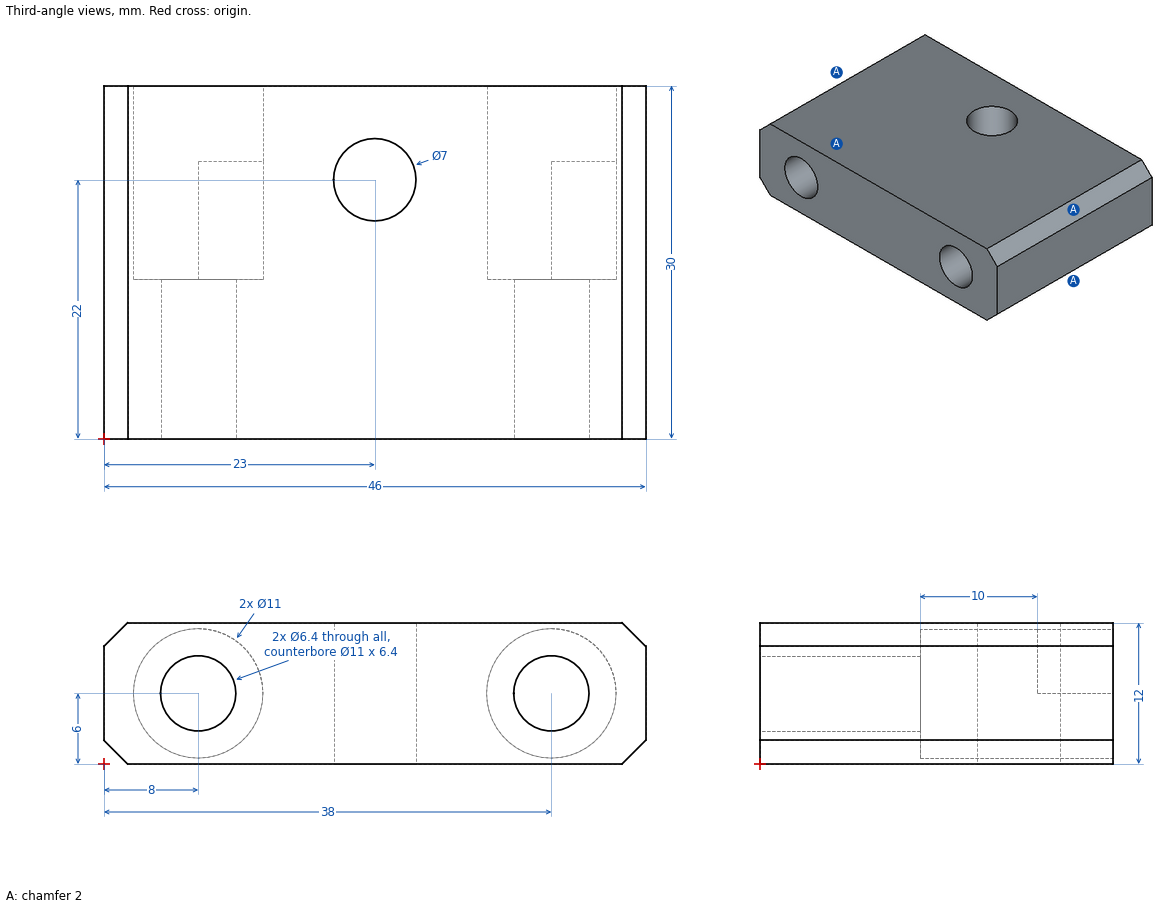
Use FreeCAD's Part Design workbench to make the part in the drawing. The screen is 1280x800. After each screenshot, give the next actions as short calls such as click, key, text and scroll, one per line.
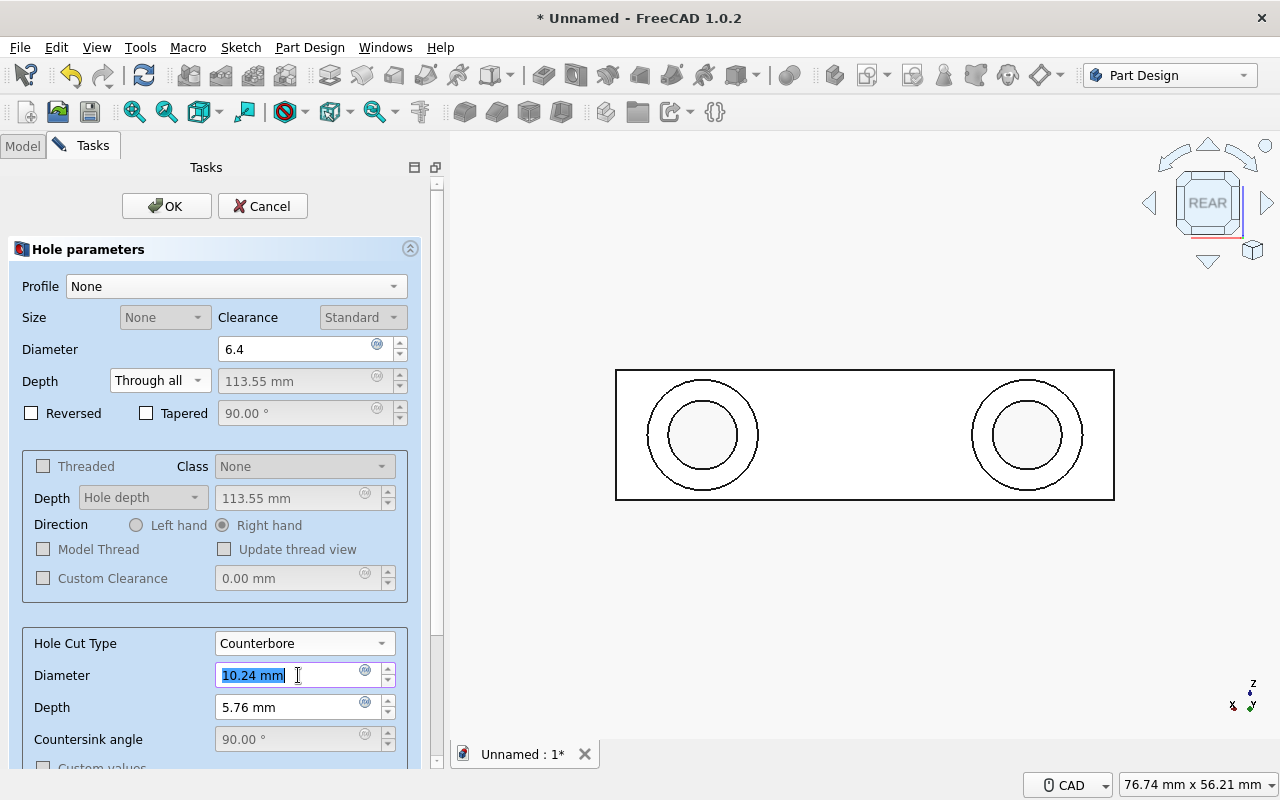
text(11)
key(Tab)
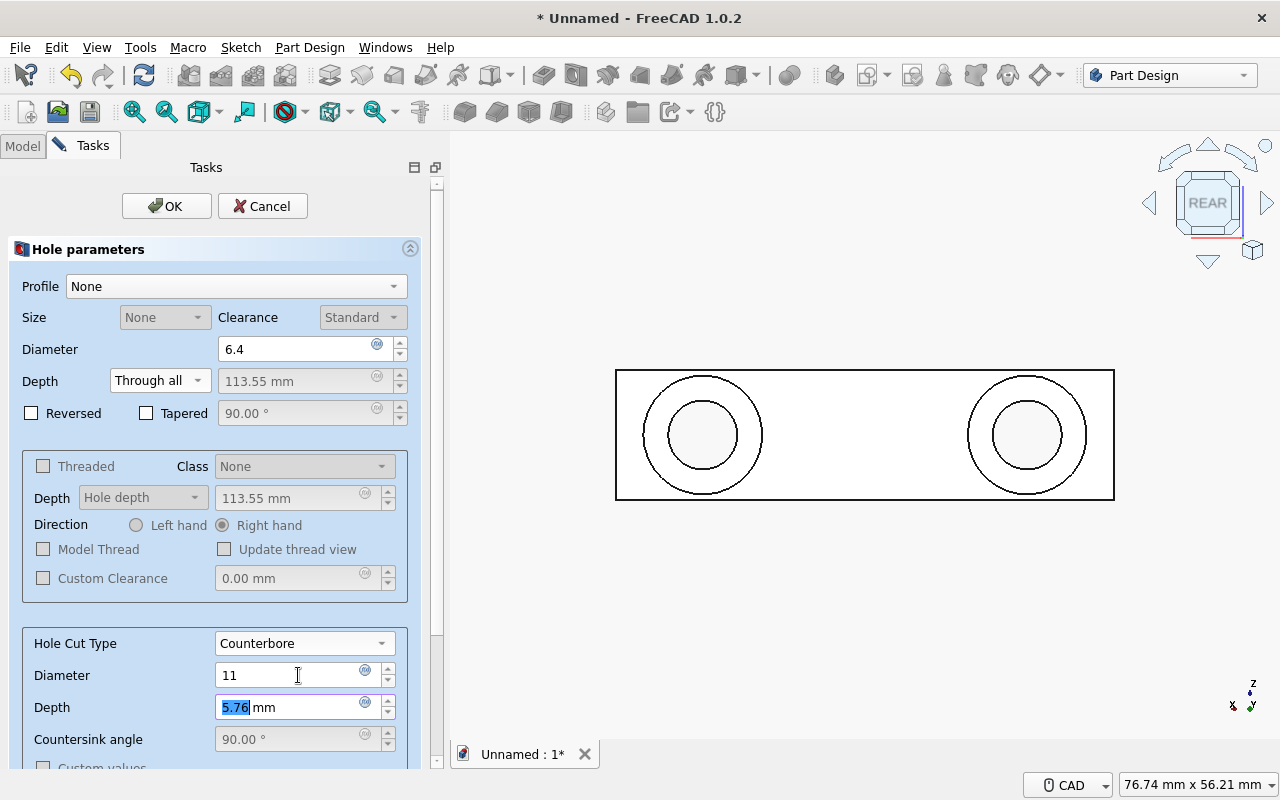
text(6.4)
key(Tab)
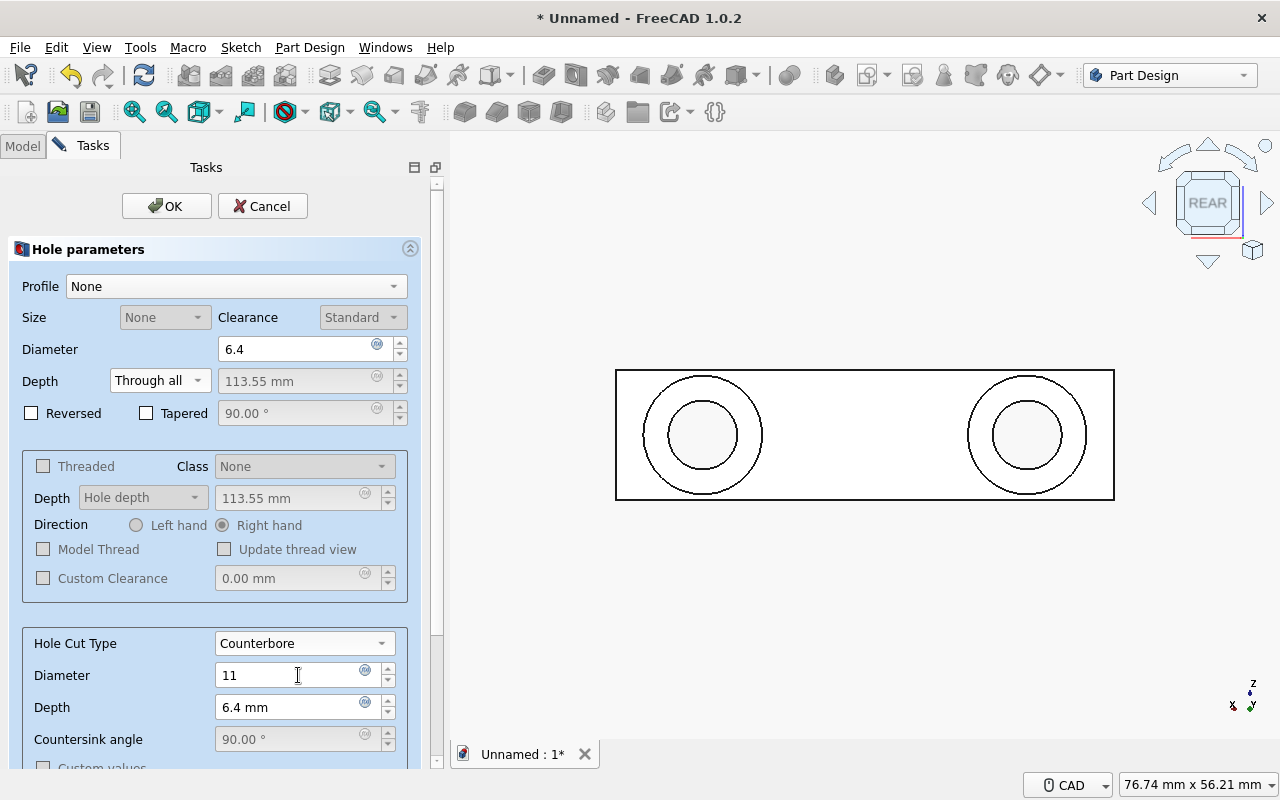
click(167, 206)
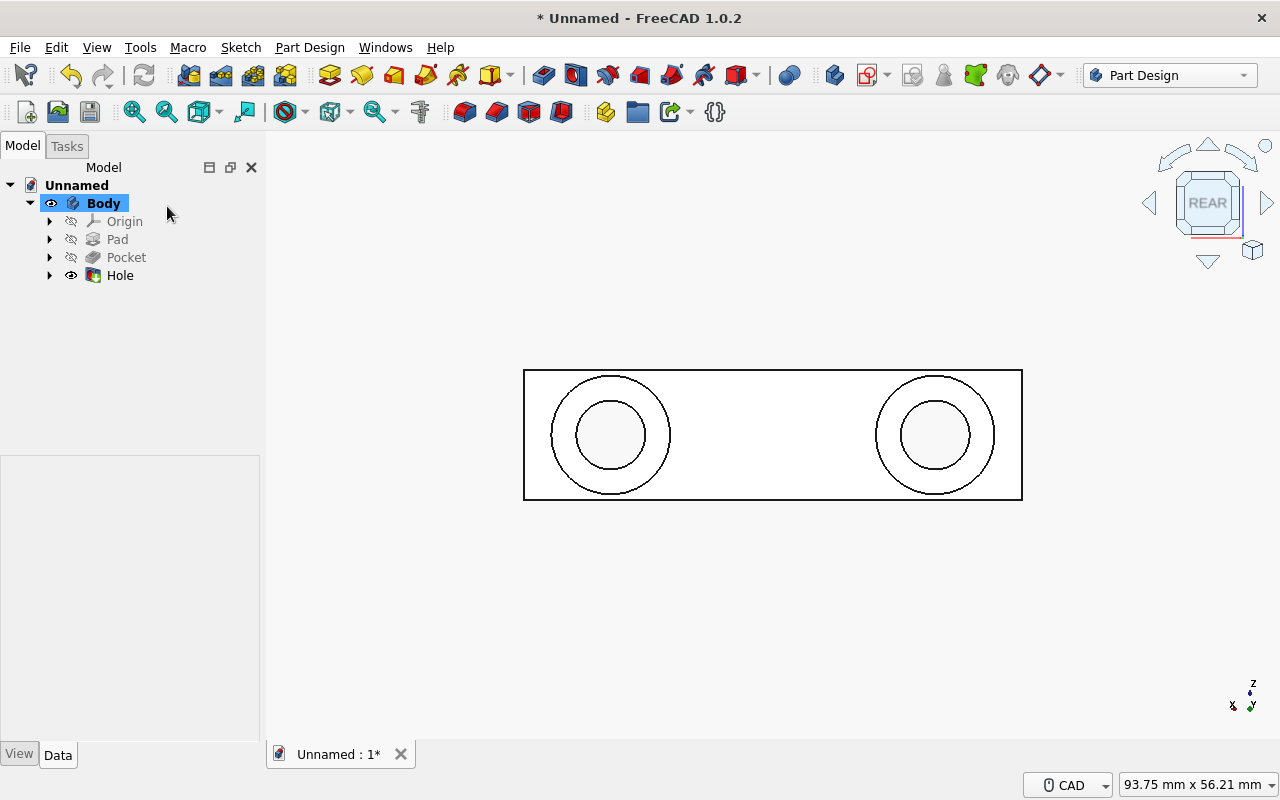
click(577, 400)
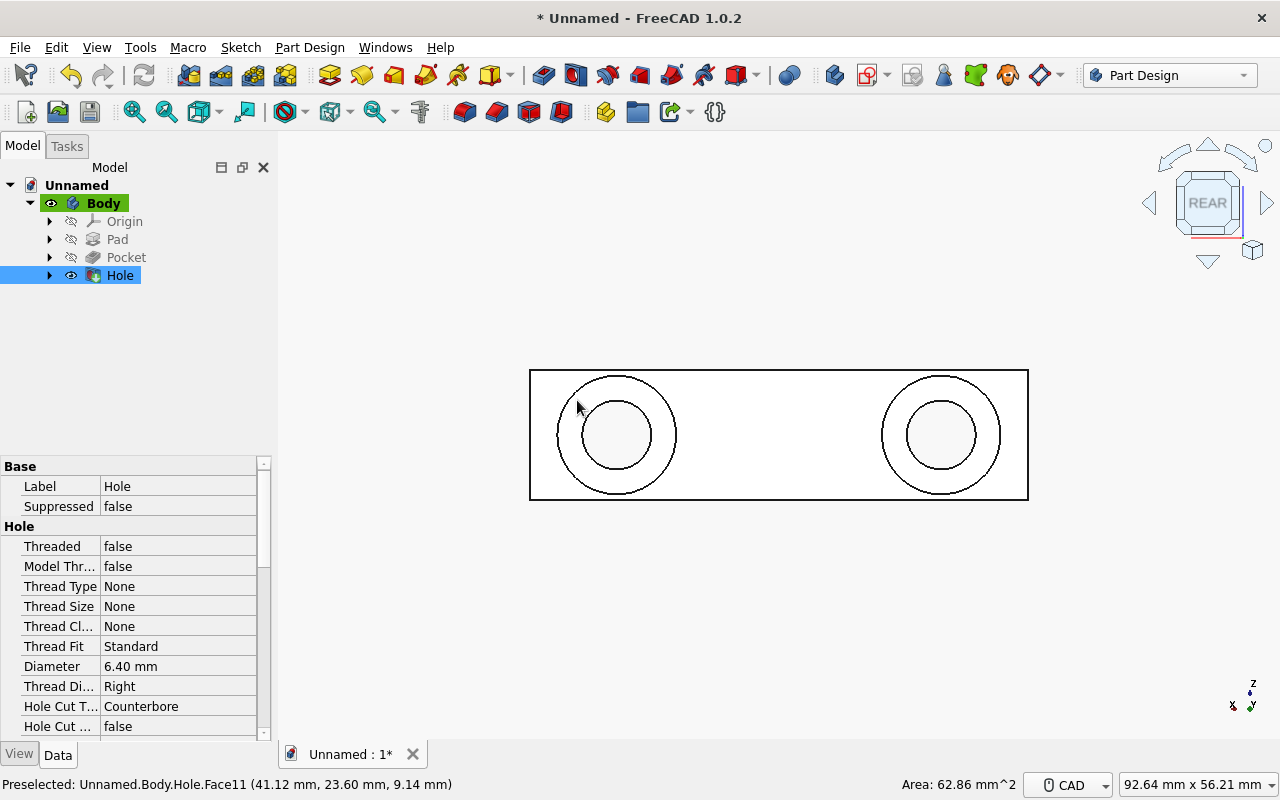
click(868, 76)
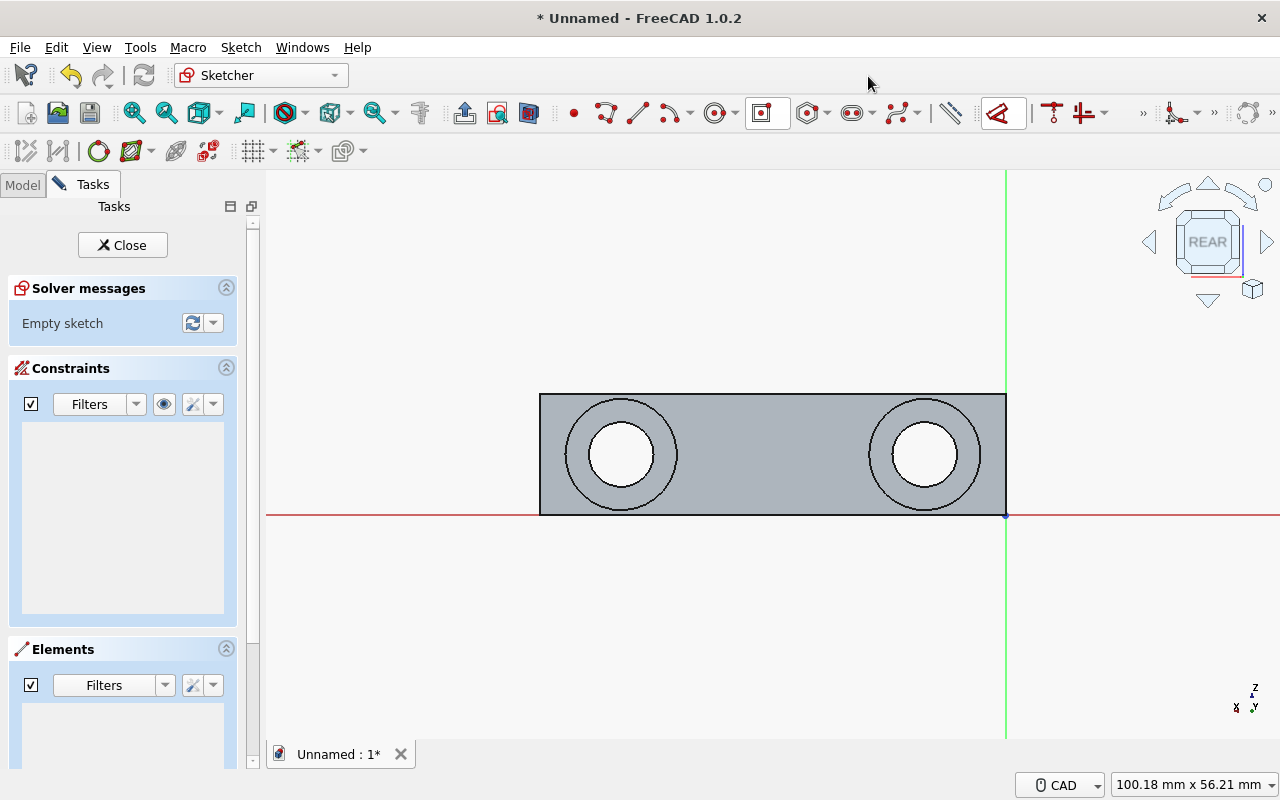
key(g)
key(c)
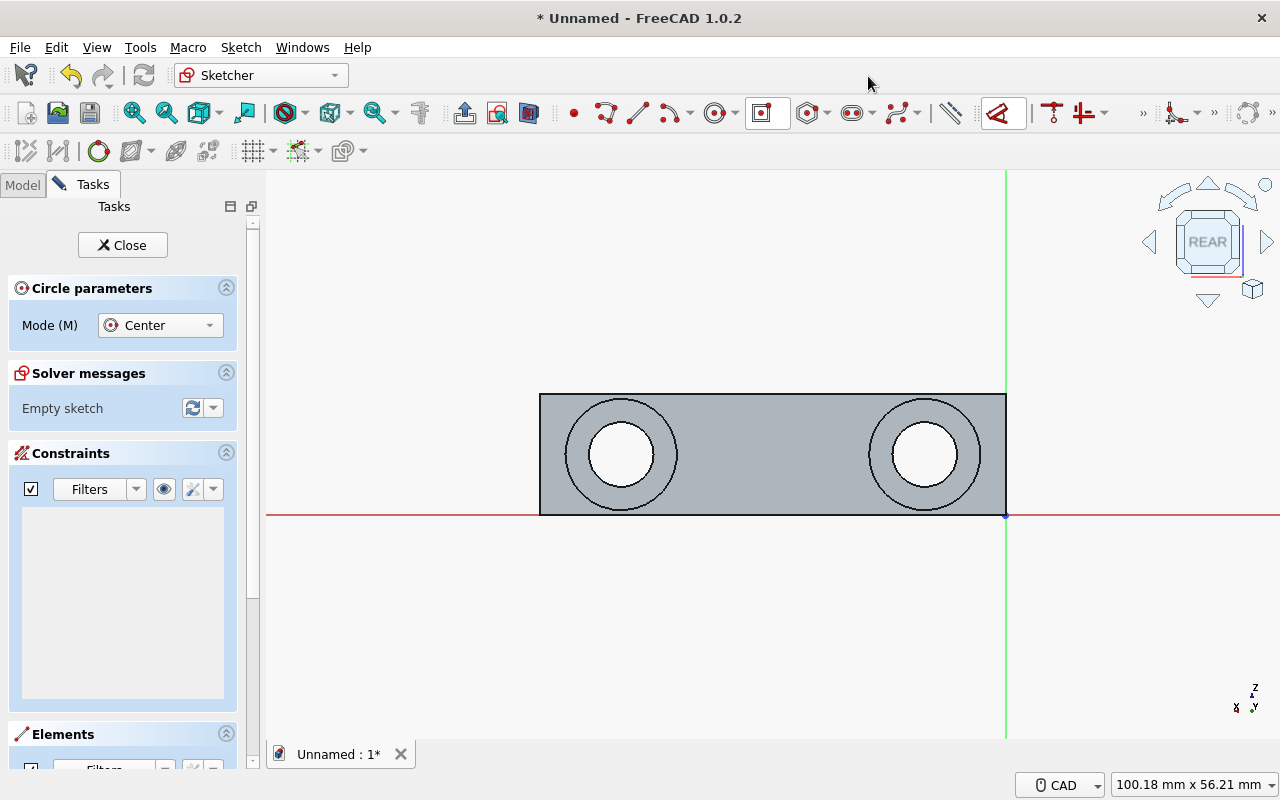
click(925, 455)
move(964, 415)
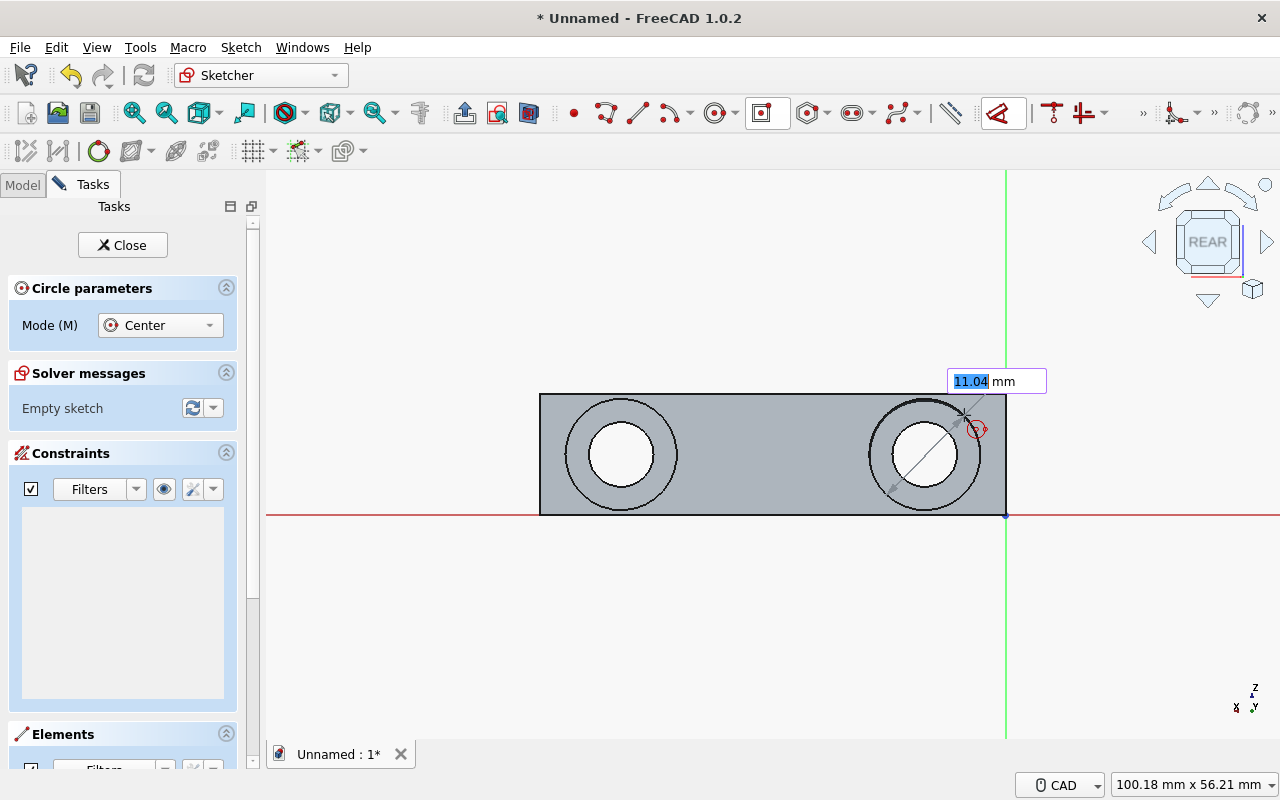
text(11)
key(Return)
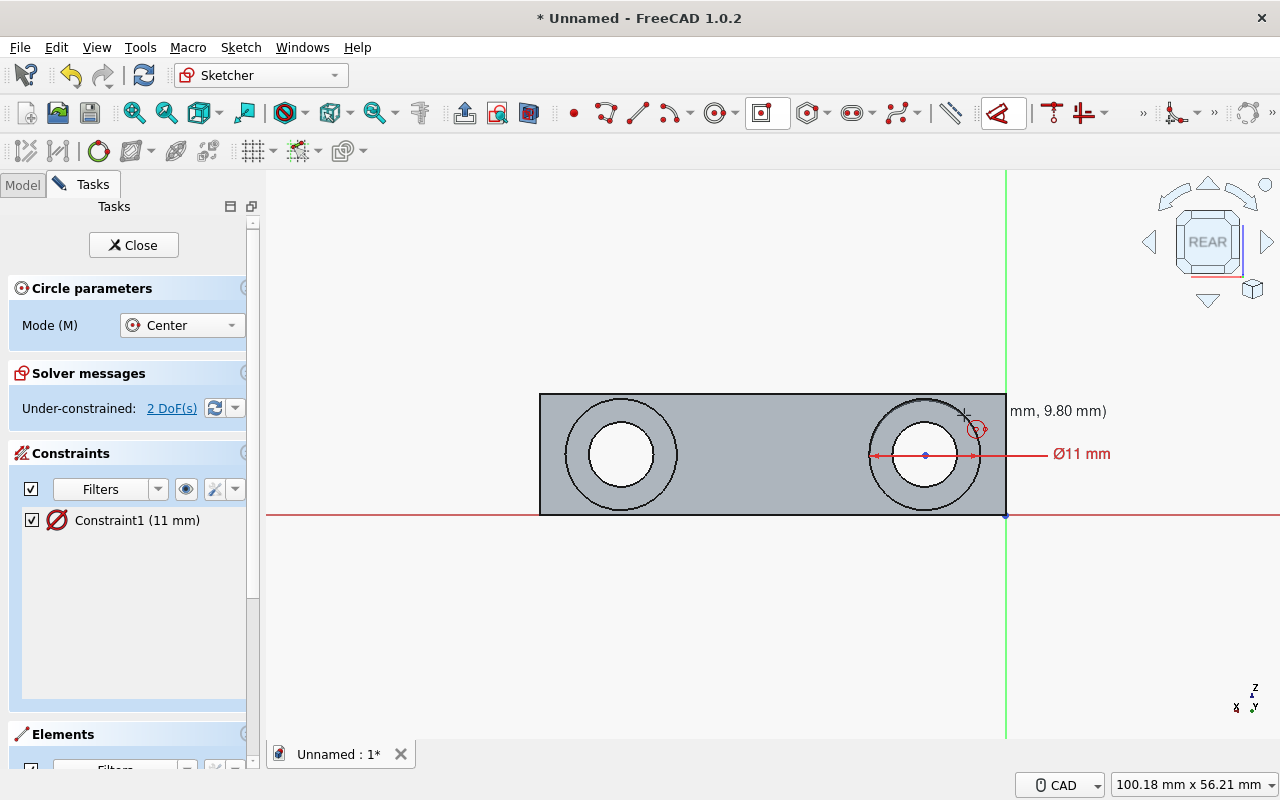
click(621, 455)
move(661, 415)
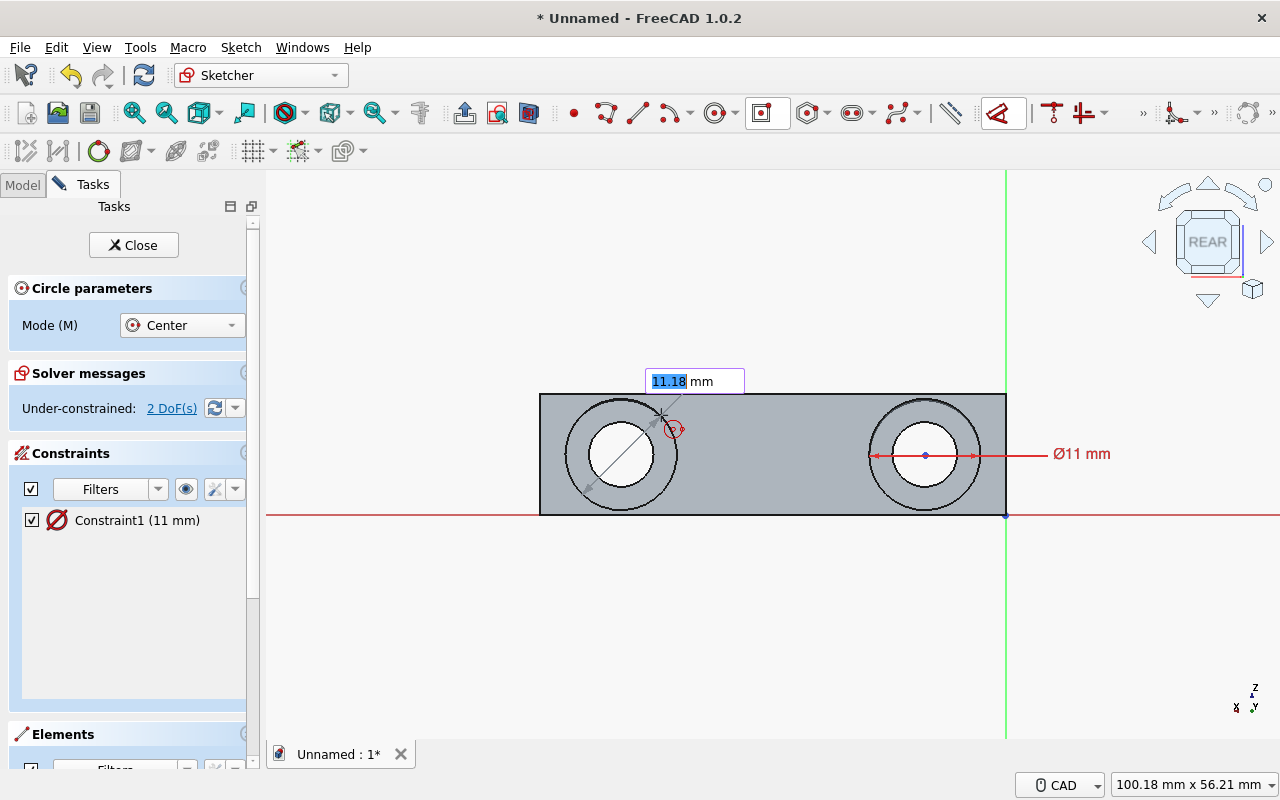
text(11)
key(Return)
key(Escape)